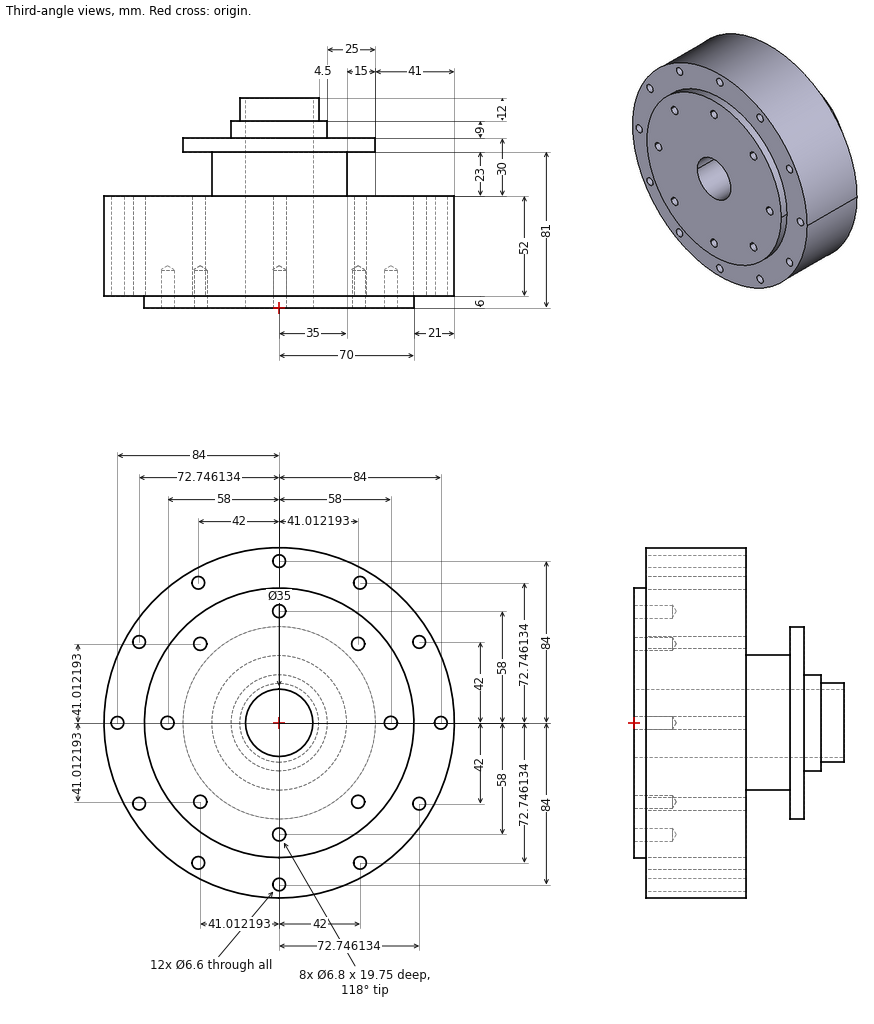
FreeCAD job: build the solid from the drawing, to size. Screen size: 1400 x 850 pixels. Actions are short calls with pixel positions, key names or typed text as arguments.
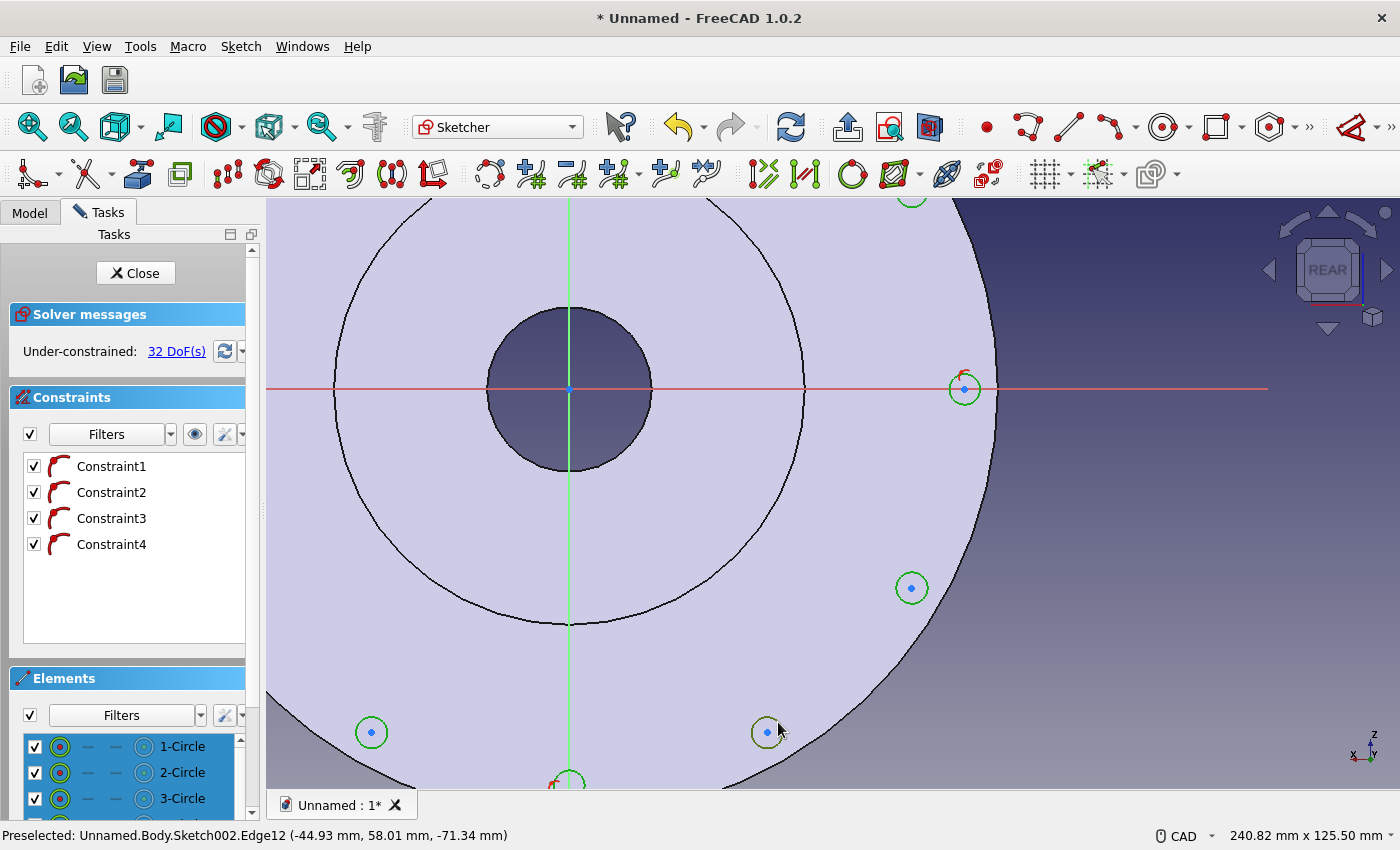
key(e)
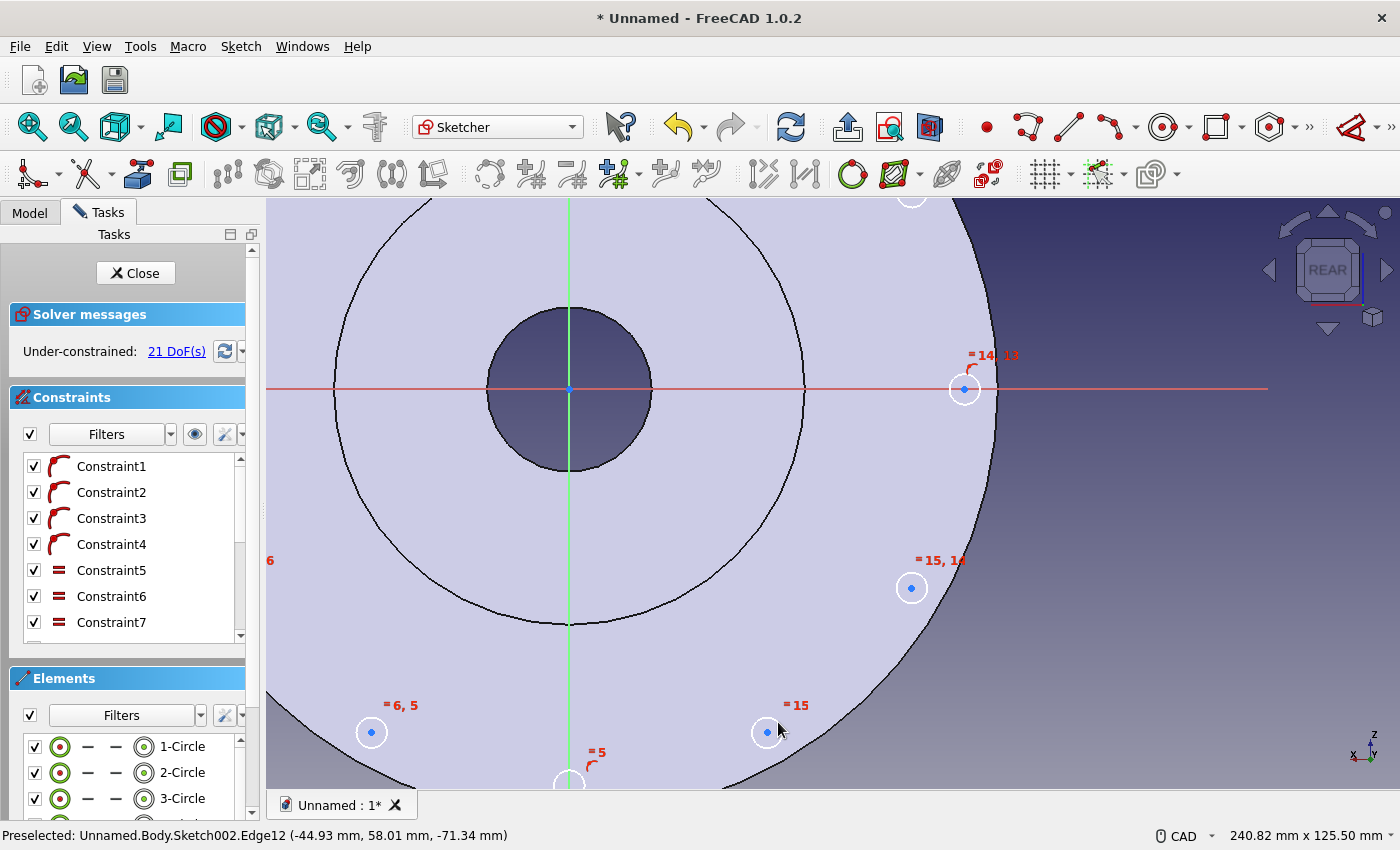
key(d)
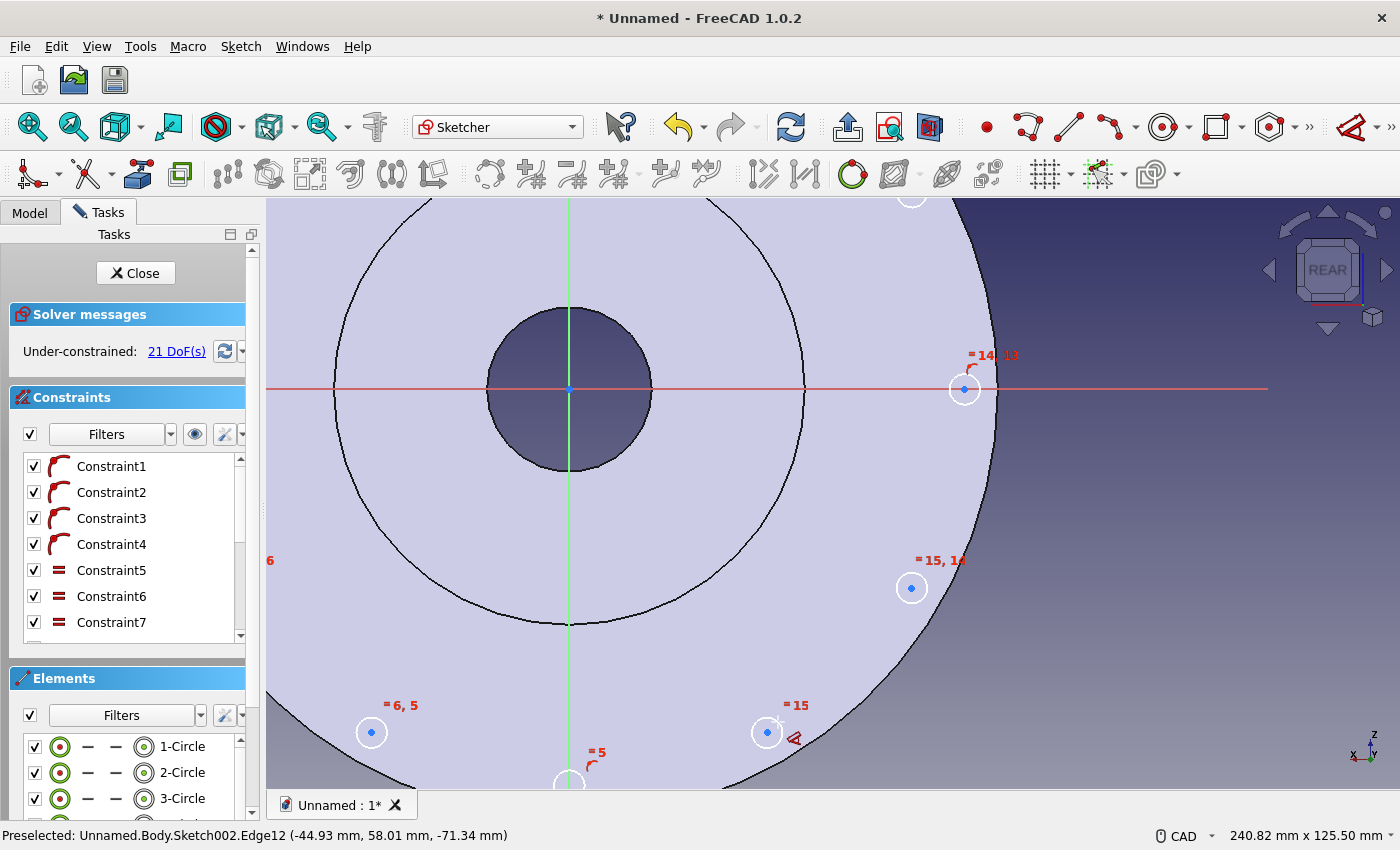
scroll(924, 578, down, 4)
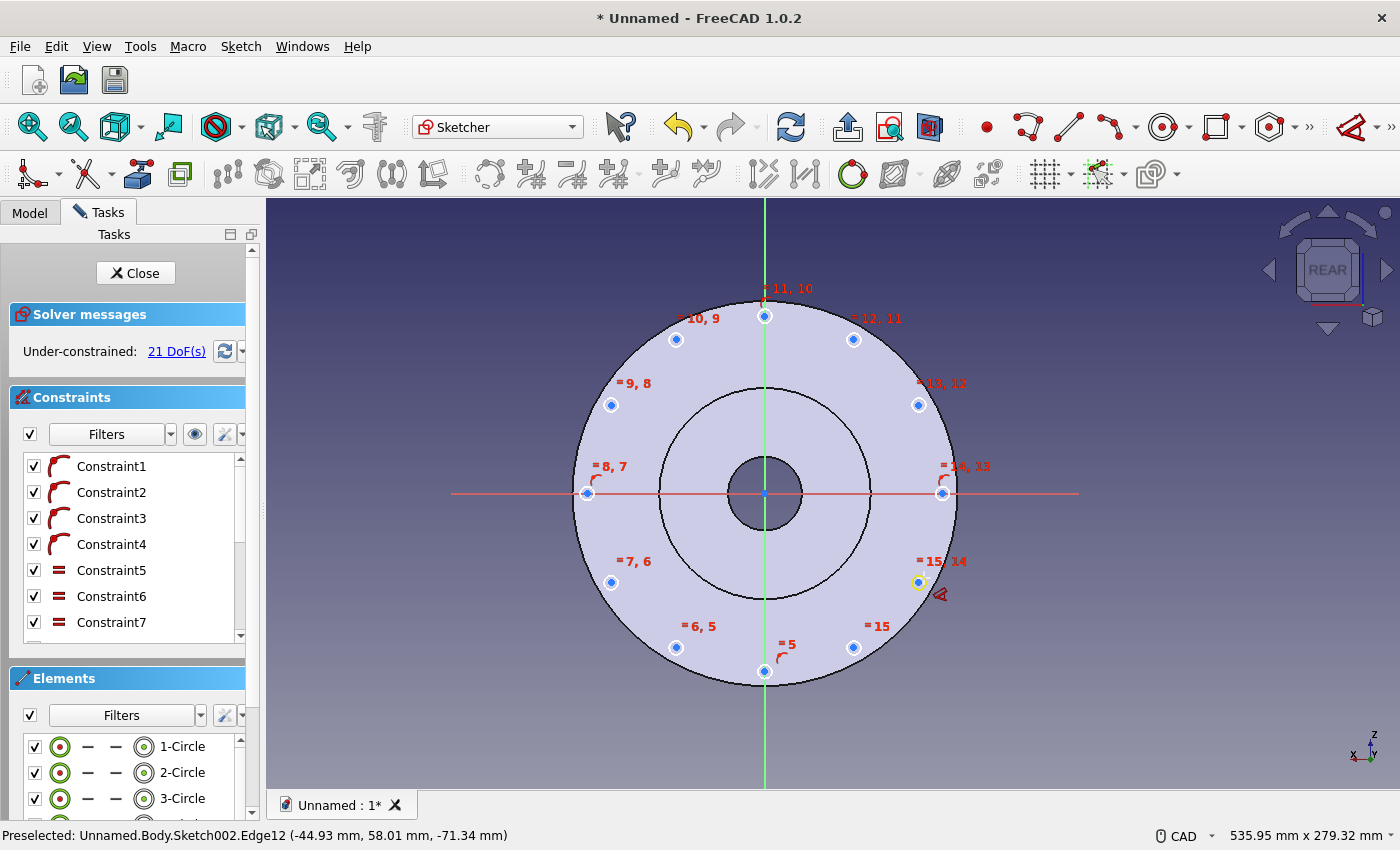
scroll(770, 667, up, 6)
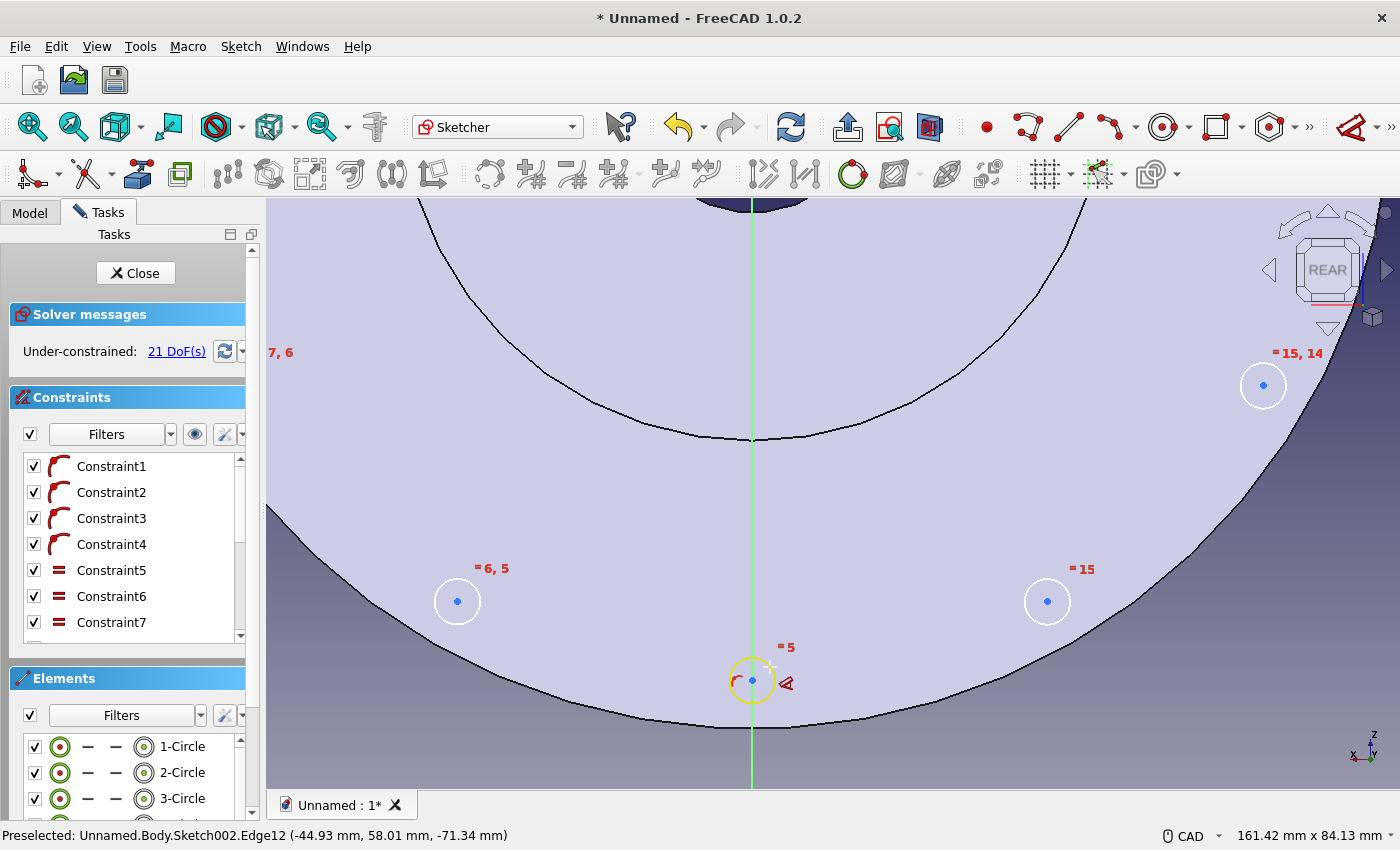
click(768, 665)
click(791, 642)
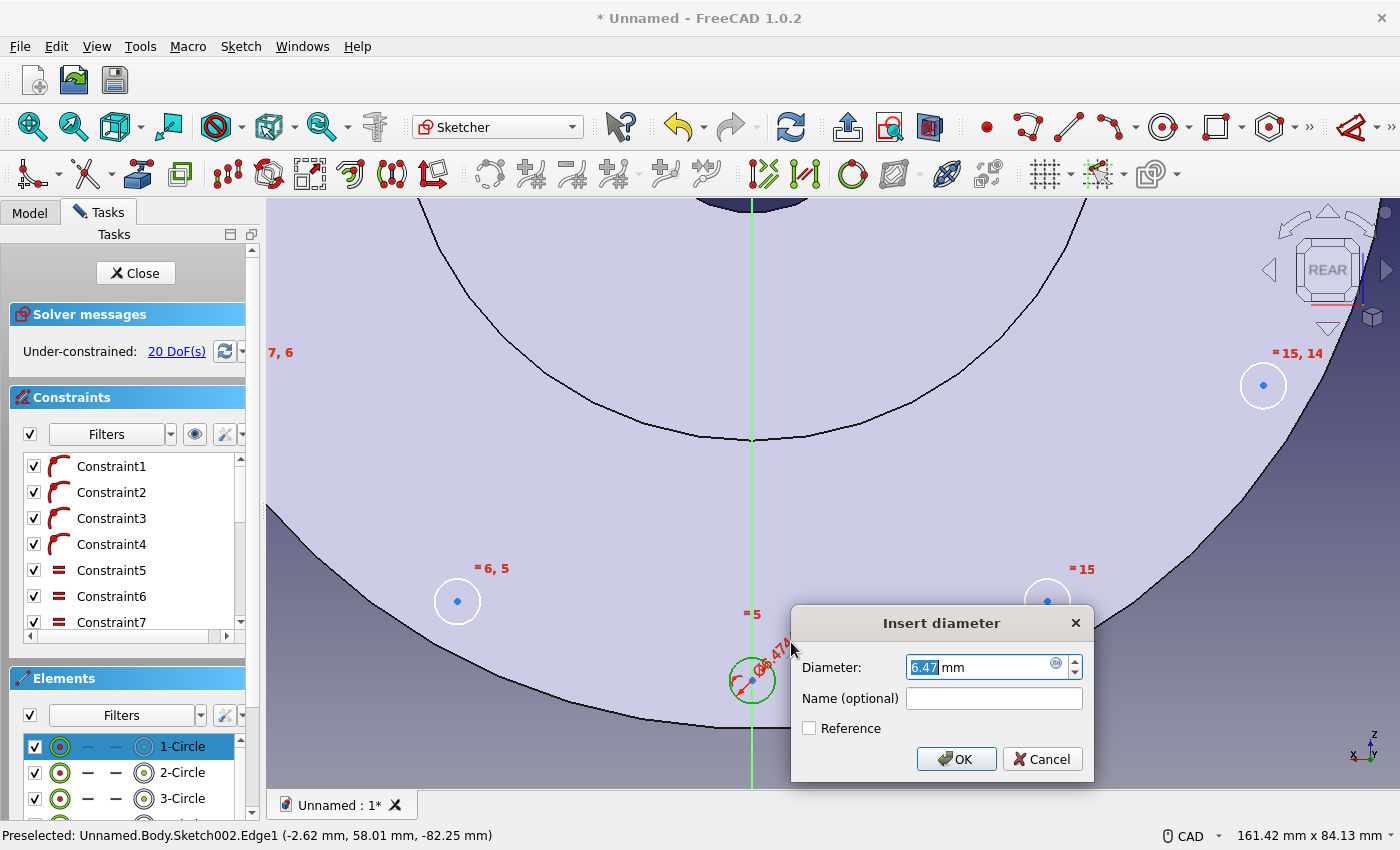
text(6.6)
key(Return)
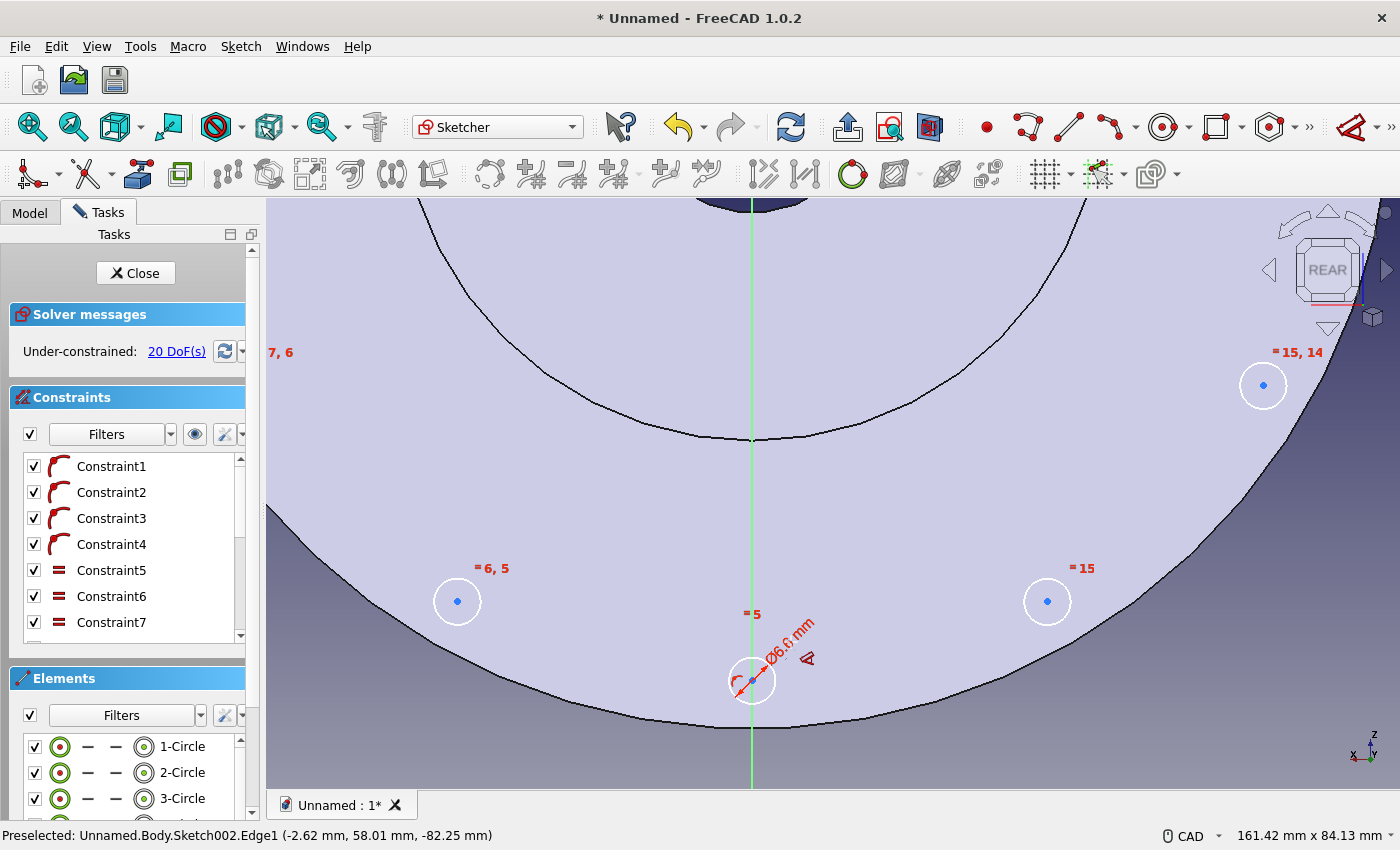
click(752, 681)
click(786, 453)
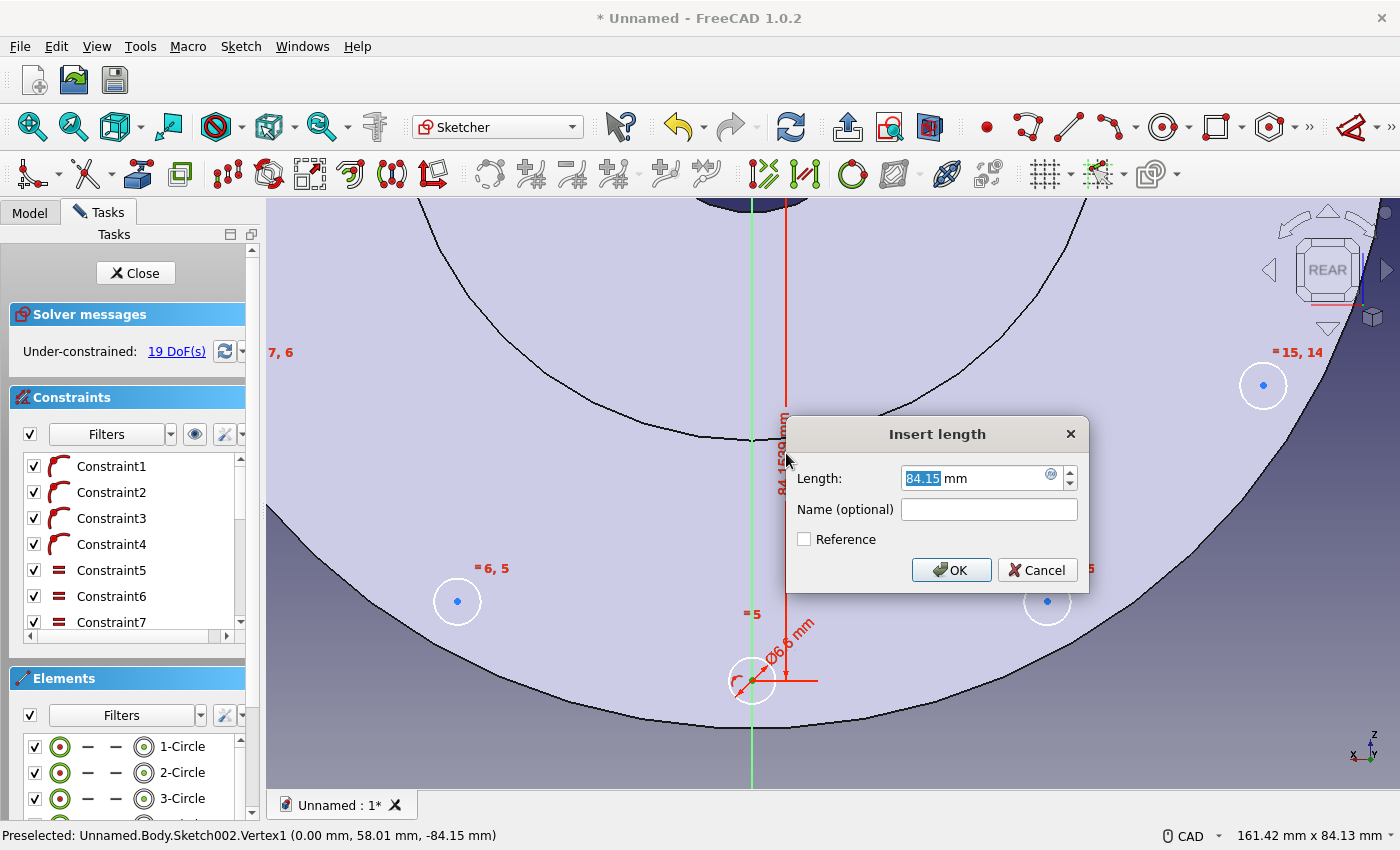
text(84)
key(Return)